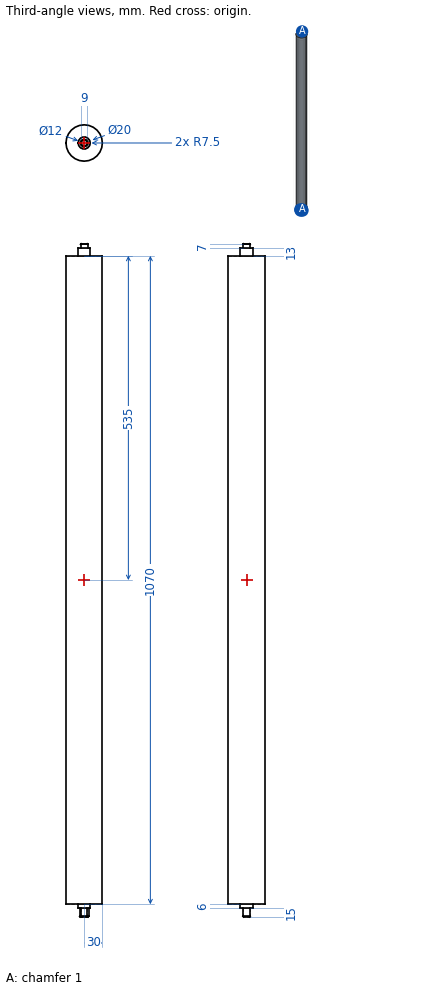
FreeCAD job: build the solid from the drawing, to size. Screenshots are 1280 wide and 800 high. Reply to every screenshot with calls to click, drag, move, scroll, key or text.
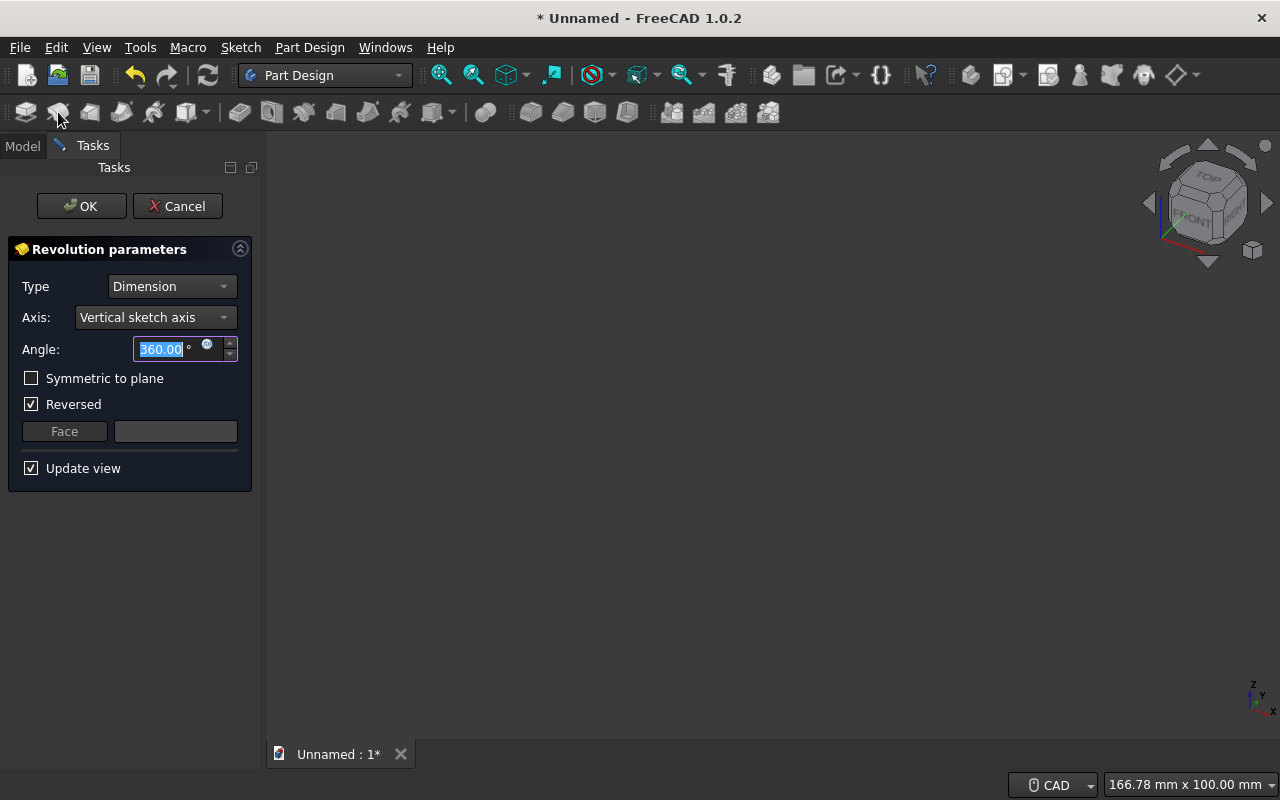
click(82, 206)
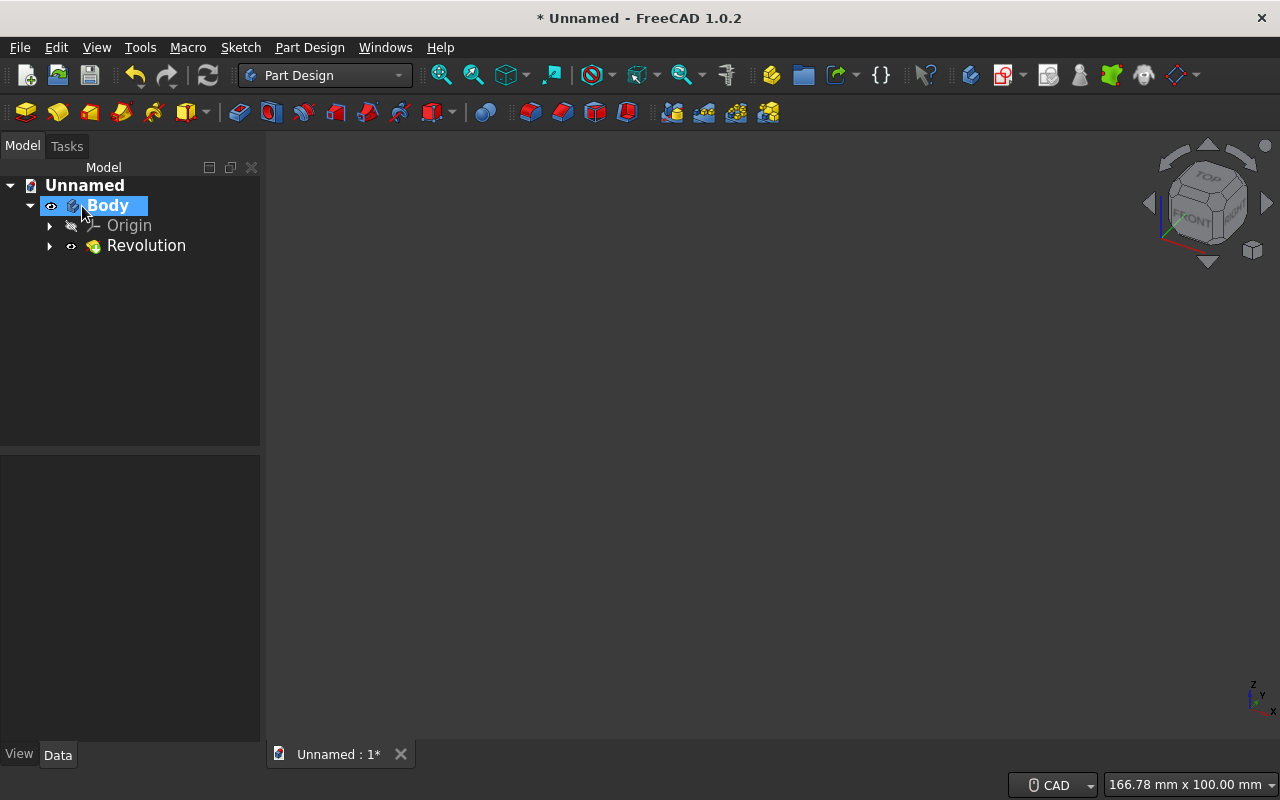
key(v)
key(f)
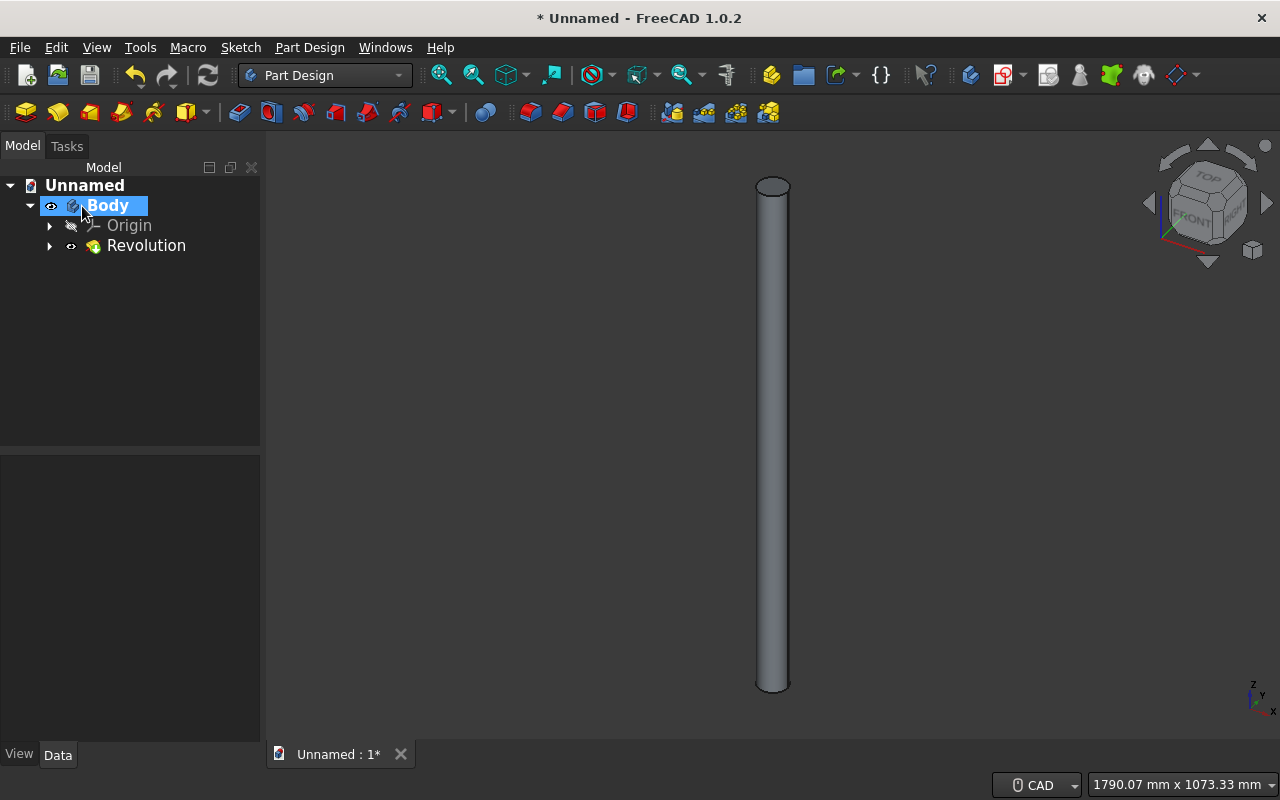
key(5)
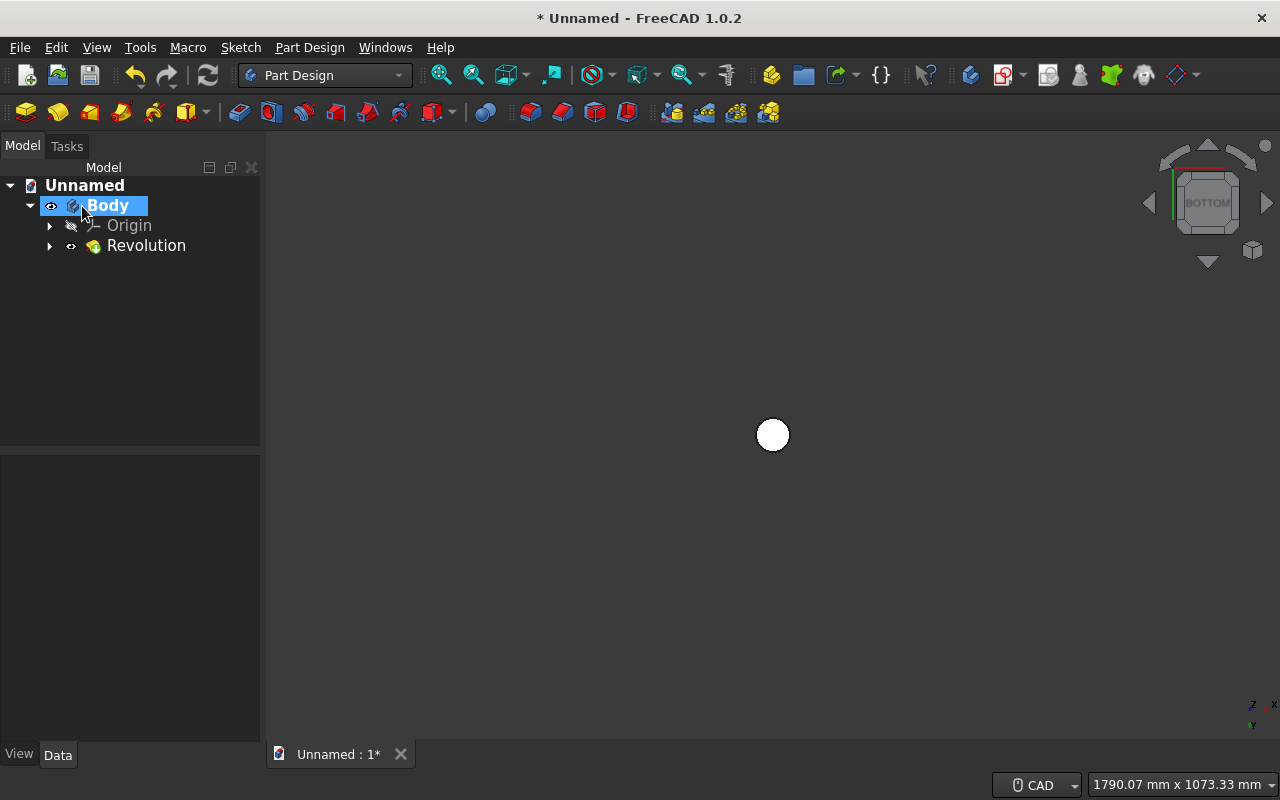
key(v)
key(f)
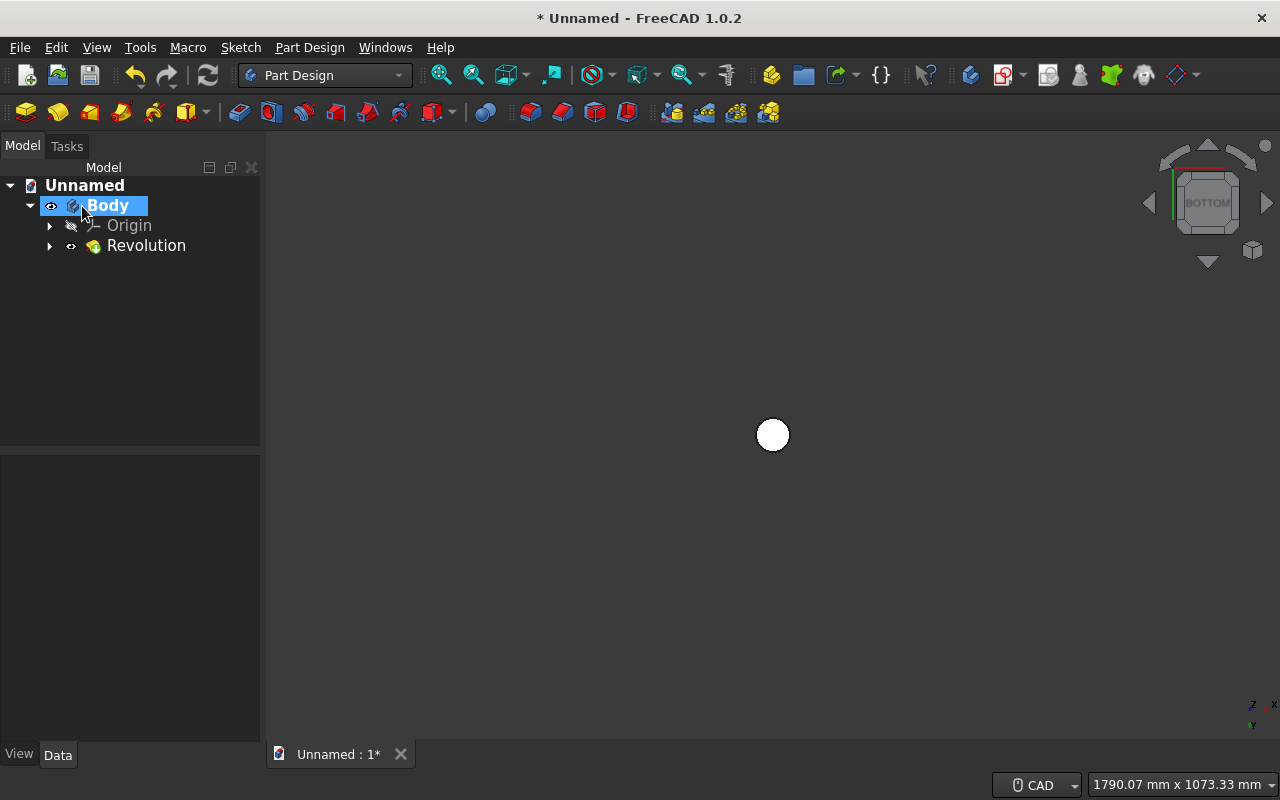
click(773, 434)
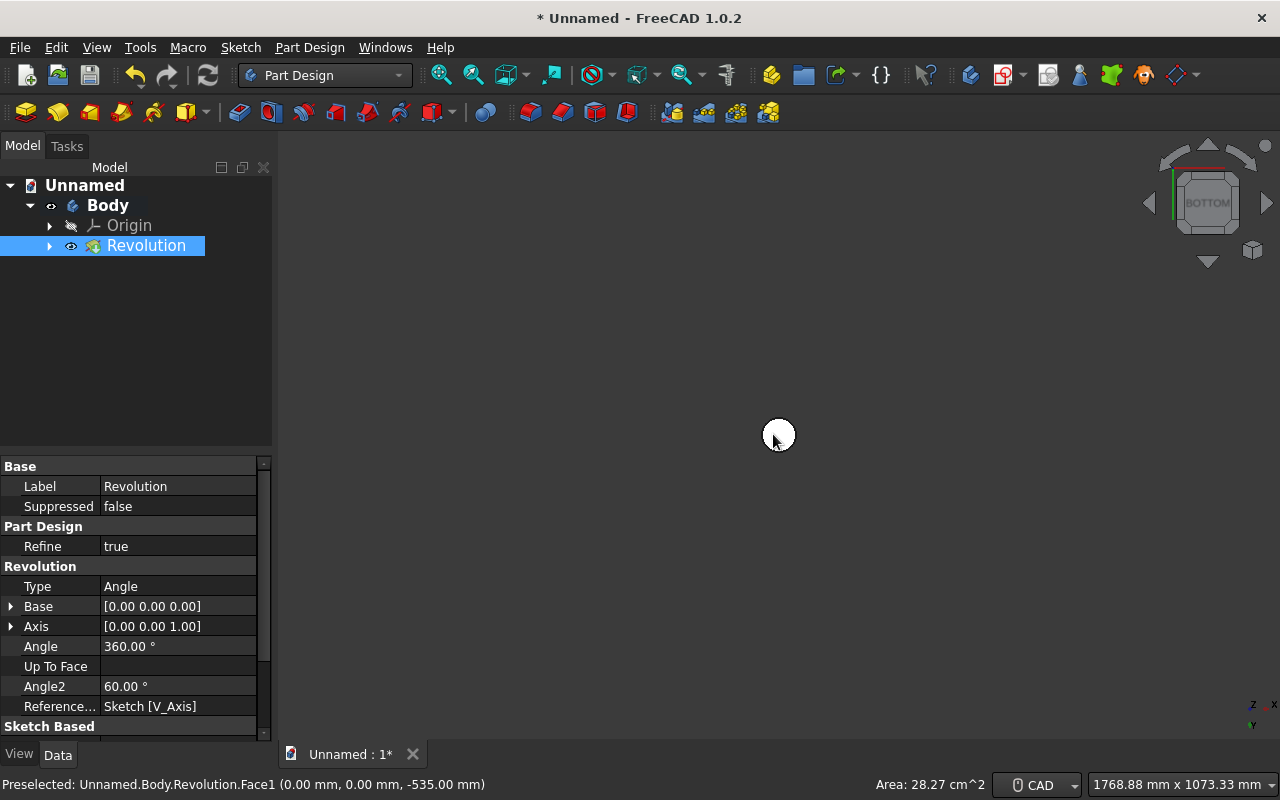
click(1004, 76)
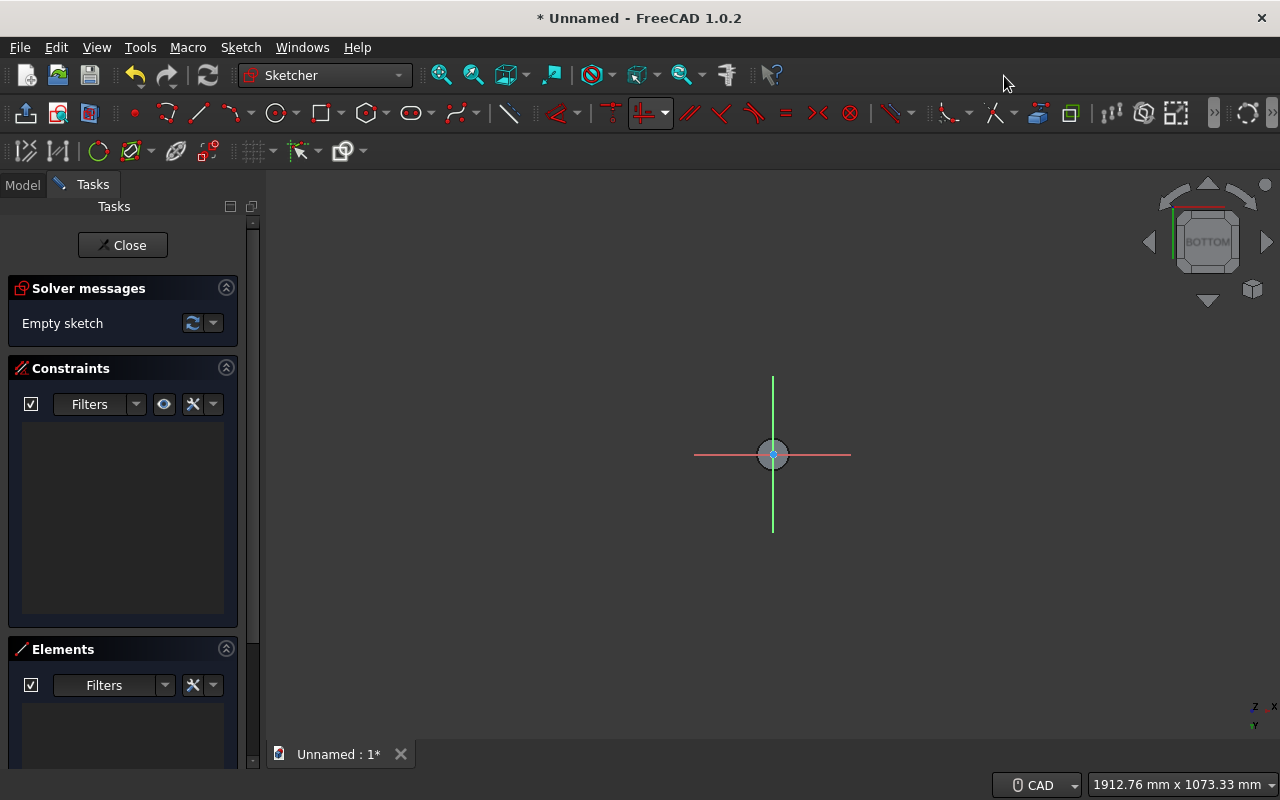
scroll(777, 454, up, 15)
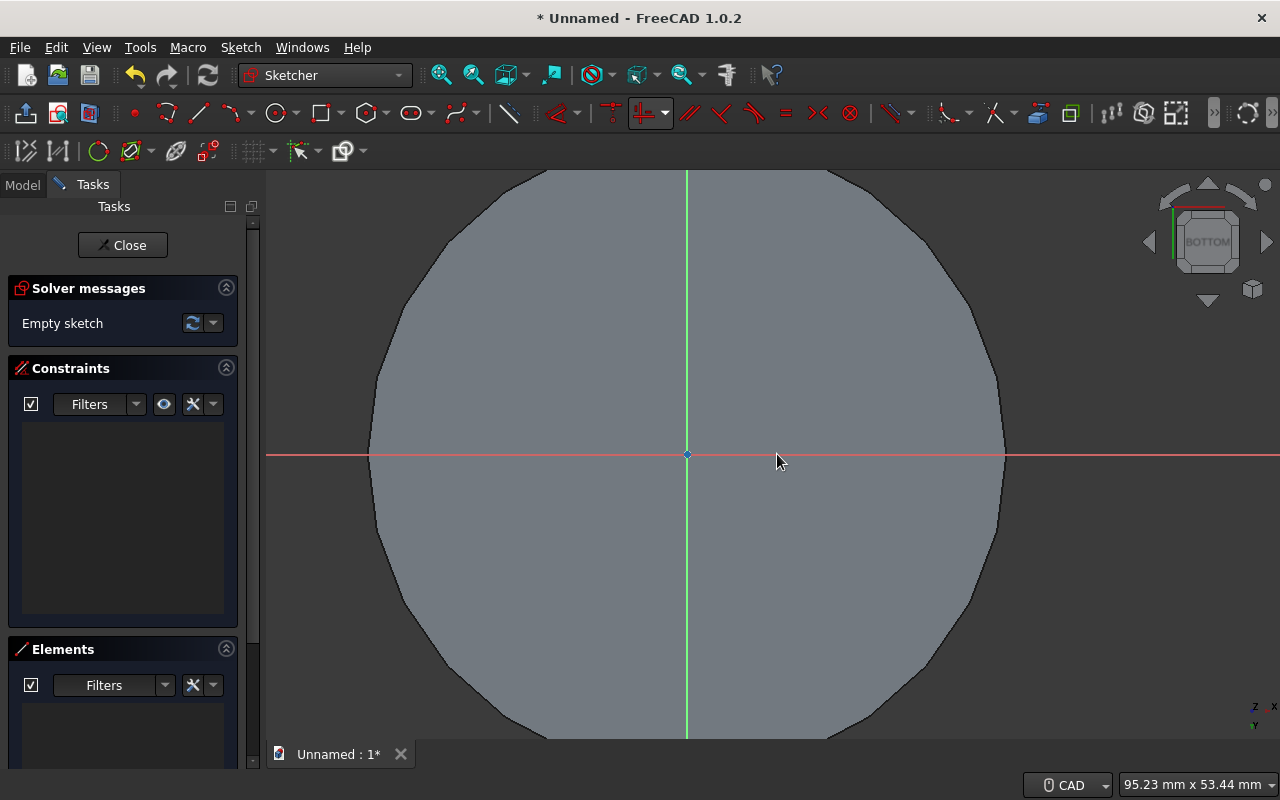
scroll(666, 454, up, 3)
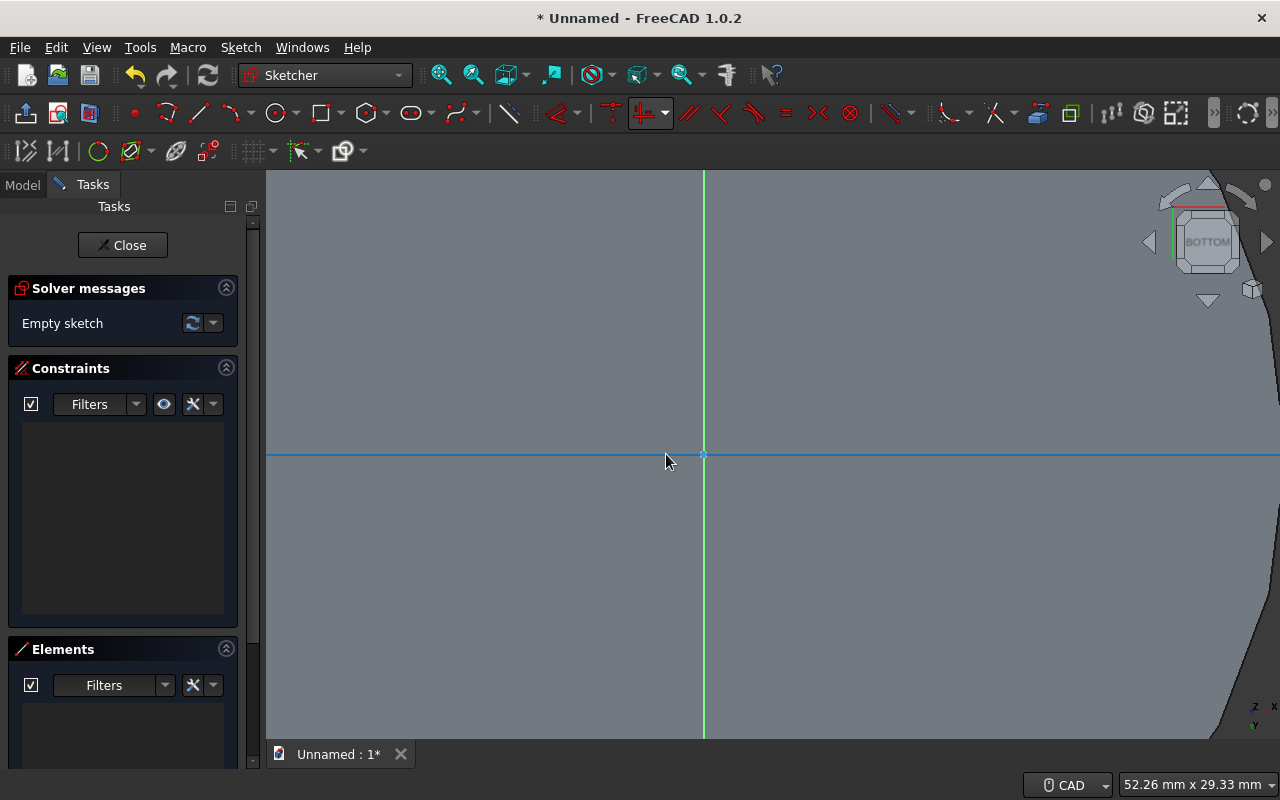
key(g)
key(c)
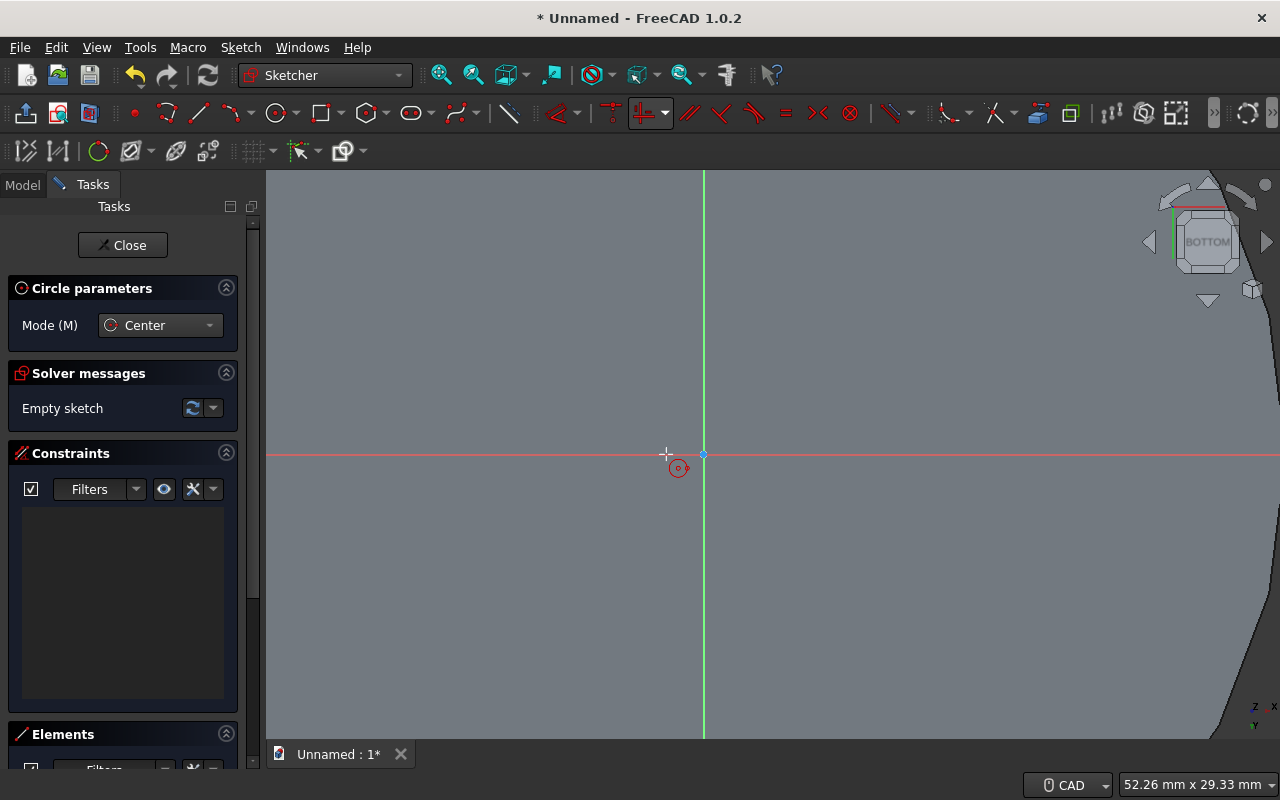
click(704, 454)
move(841, 317)